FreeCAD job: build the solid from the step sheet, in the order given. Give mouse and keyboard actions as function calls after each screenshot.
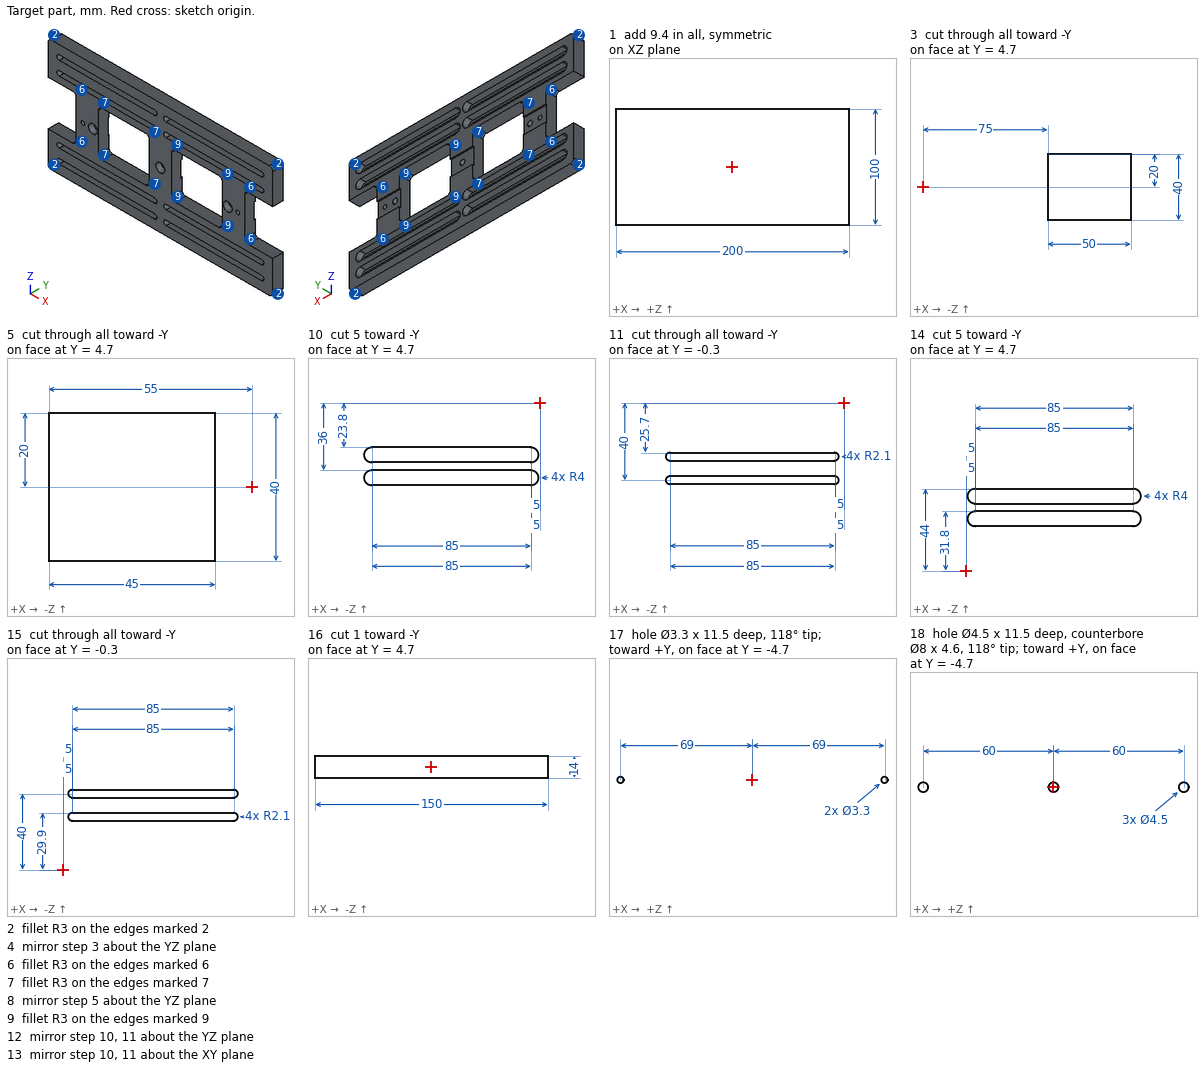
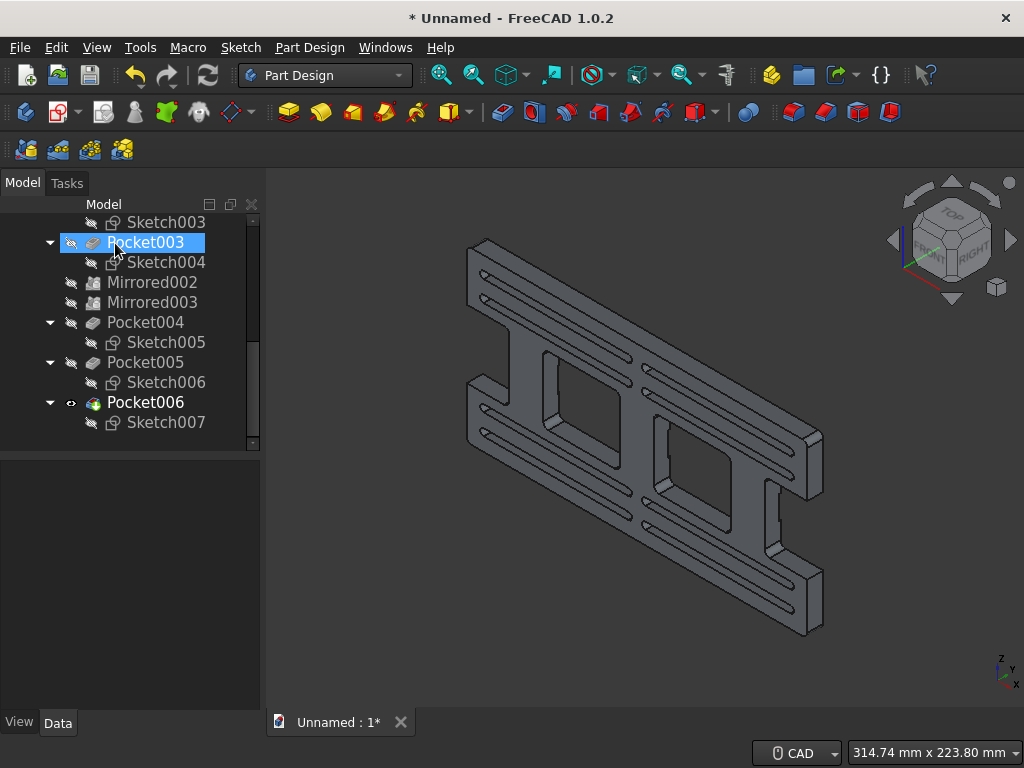
click(637, 469)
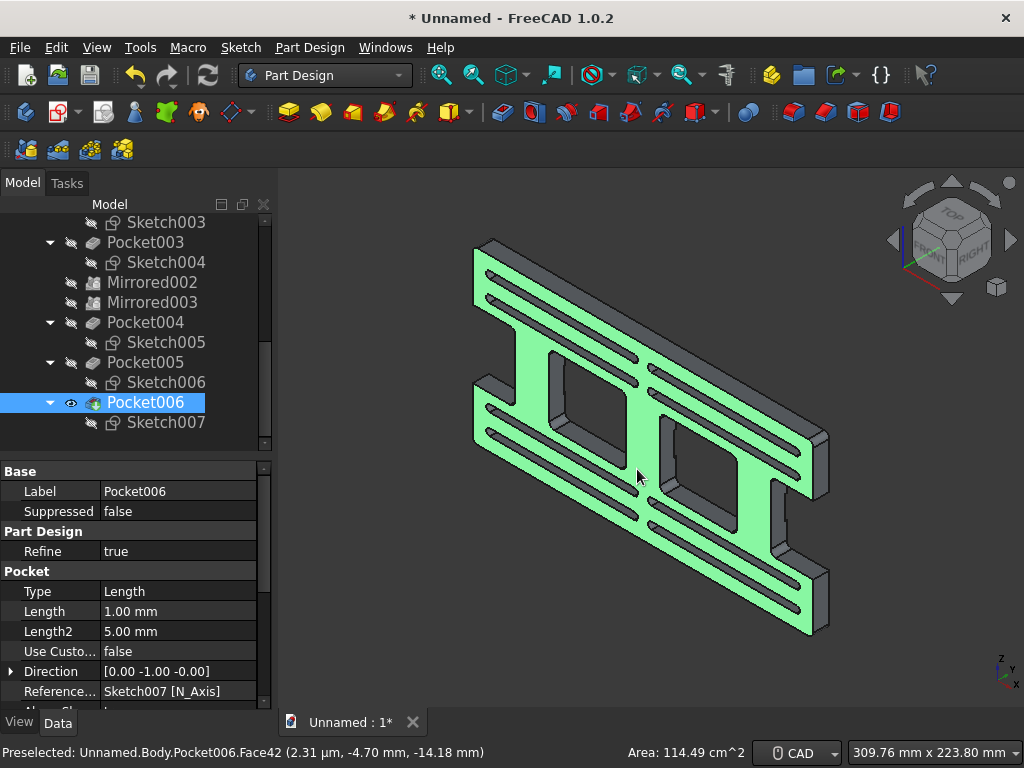
click(58, 112)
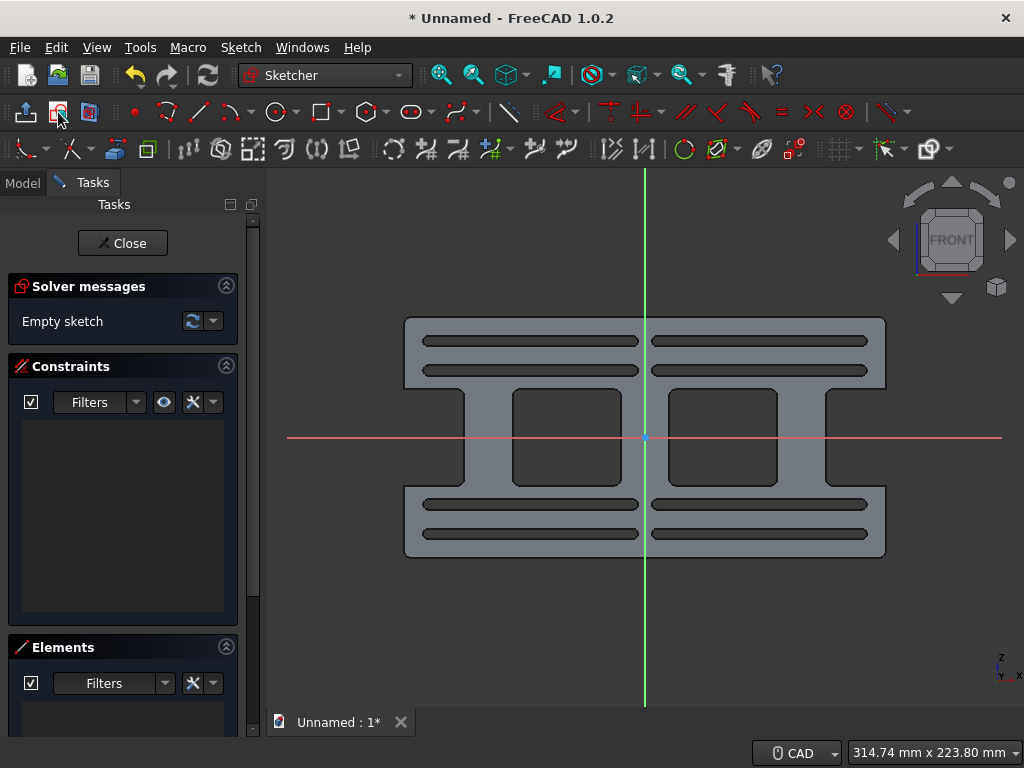
key(g)
key(c)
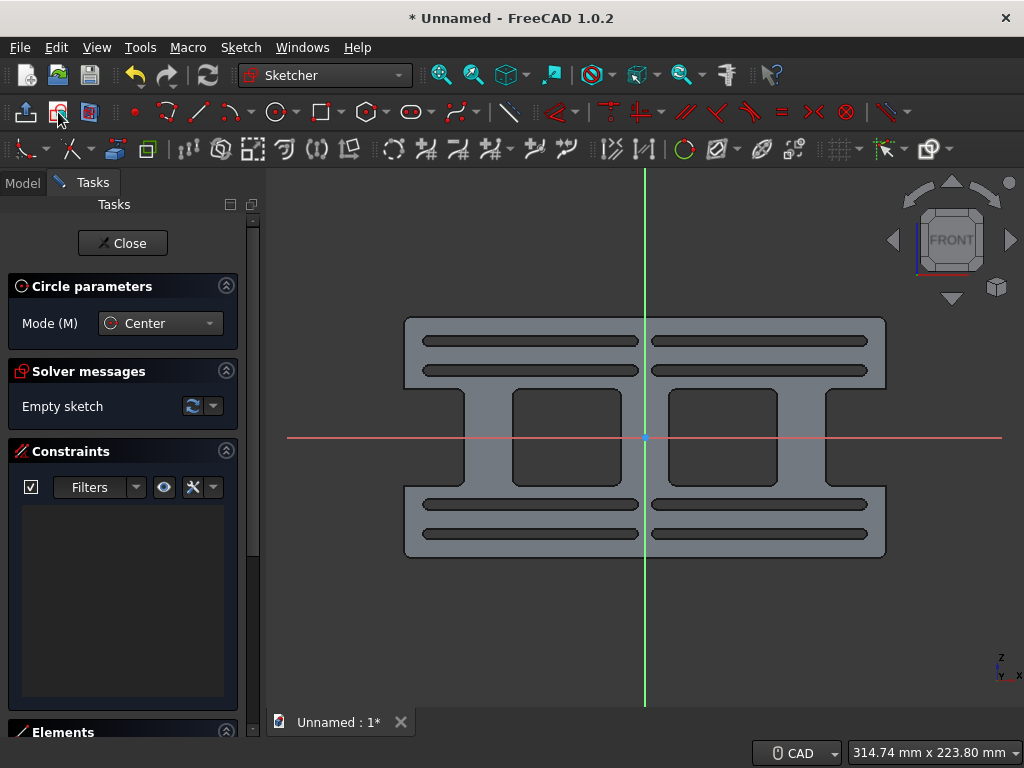
scroll(811, 438, up, 9)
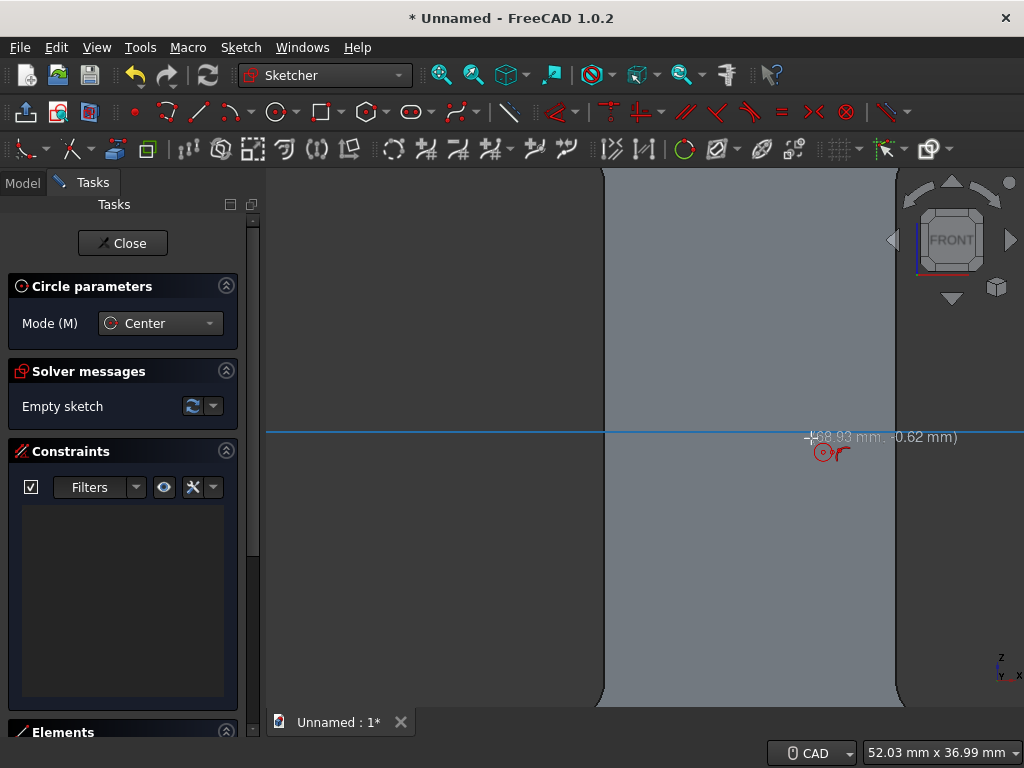
scroll(772, 439, down, 8)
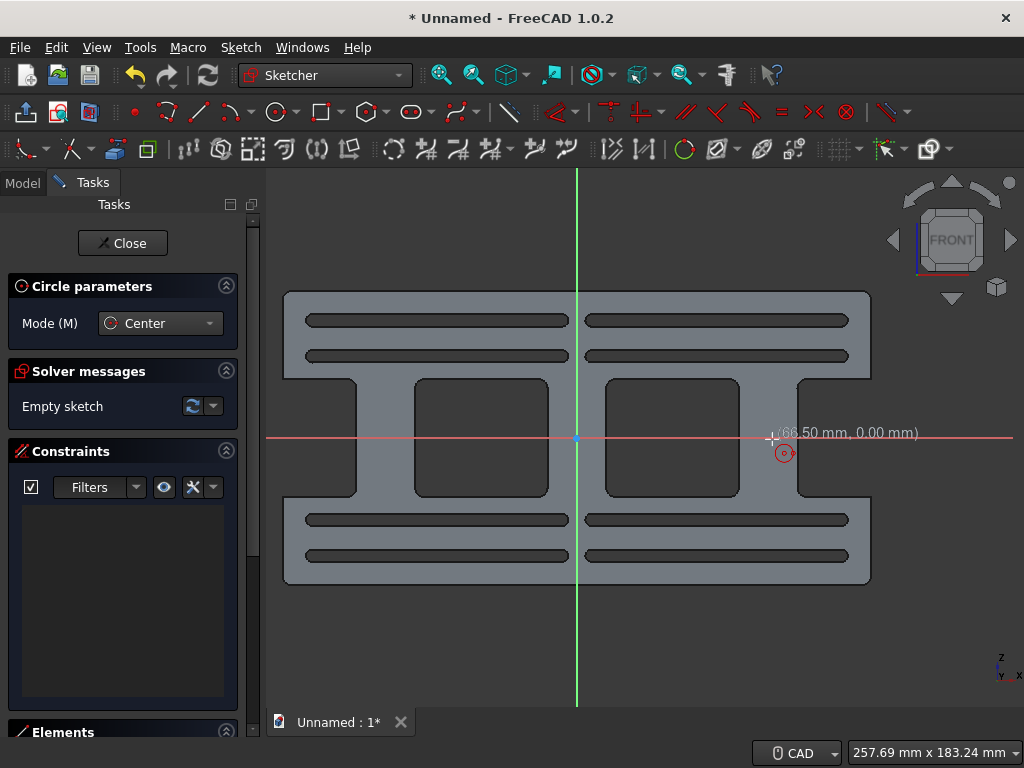
click(780, 438)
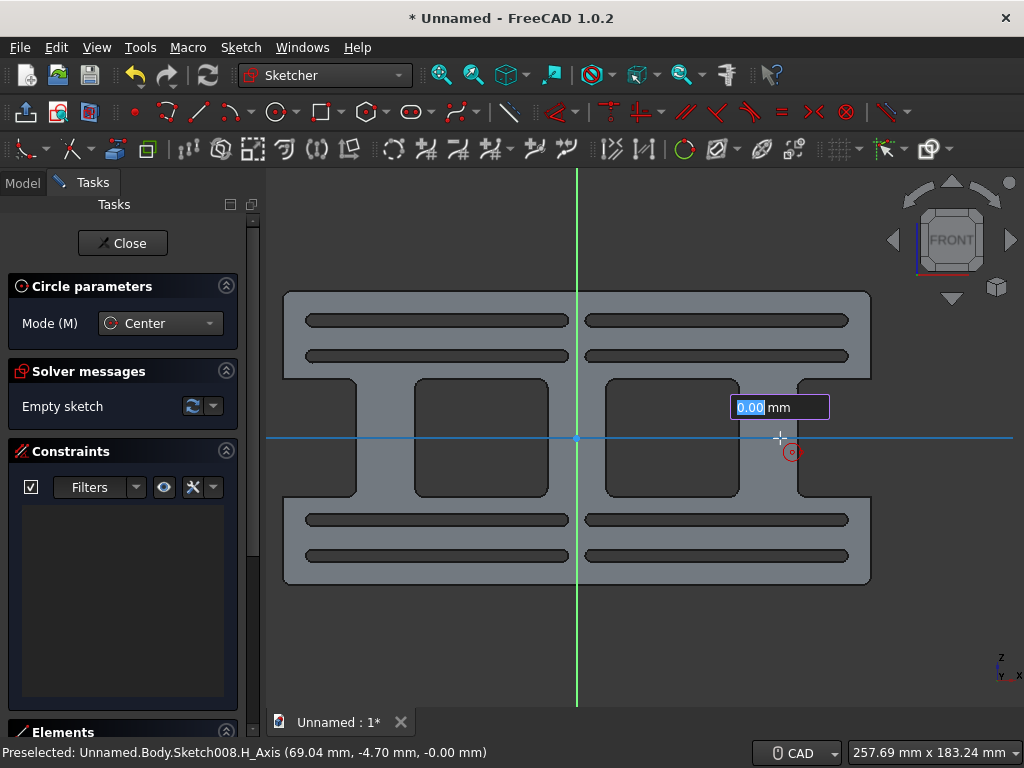
scroll(778, 443, up, 7)
move(777, 440)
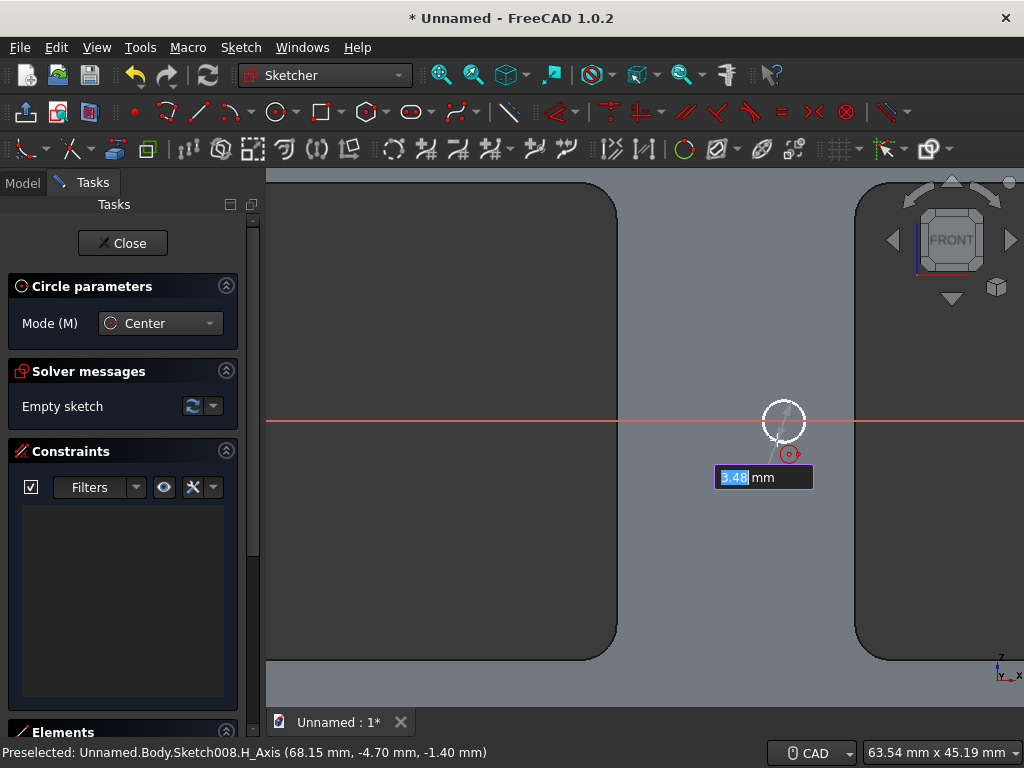
text(3.3)
key(Return)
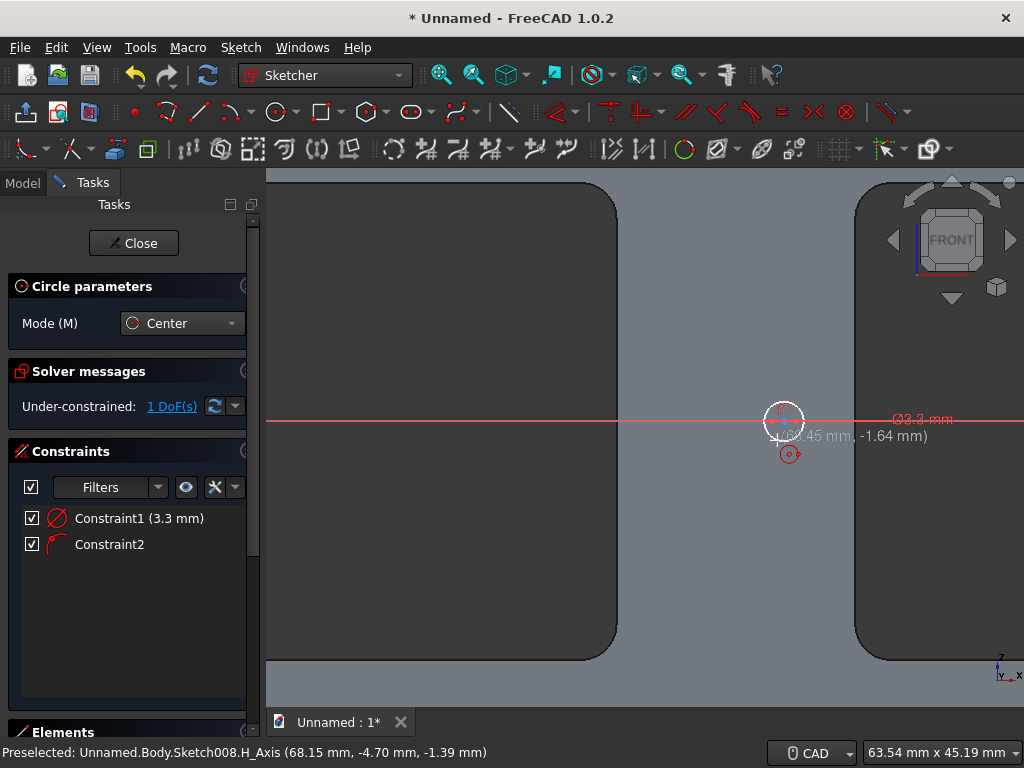
scroll(778, 443, down, 7)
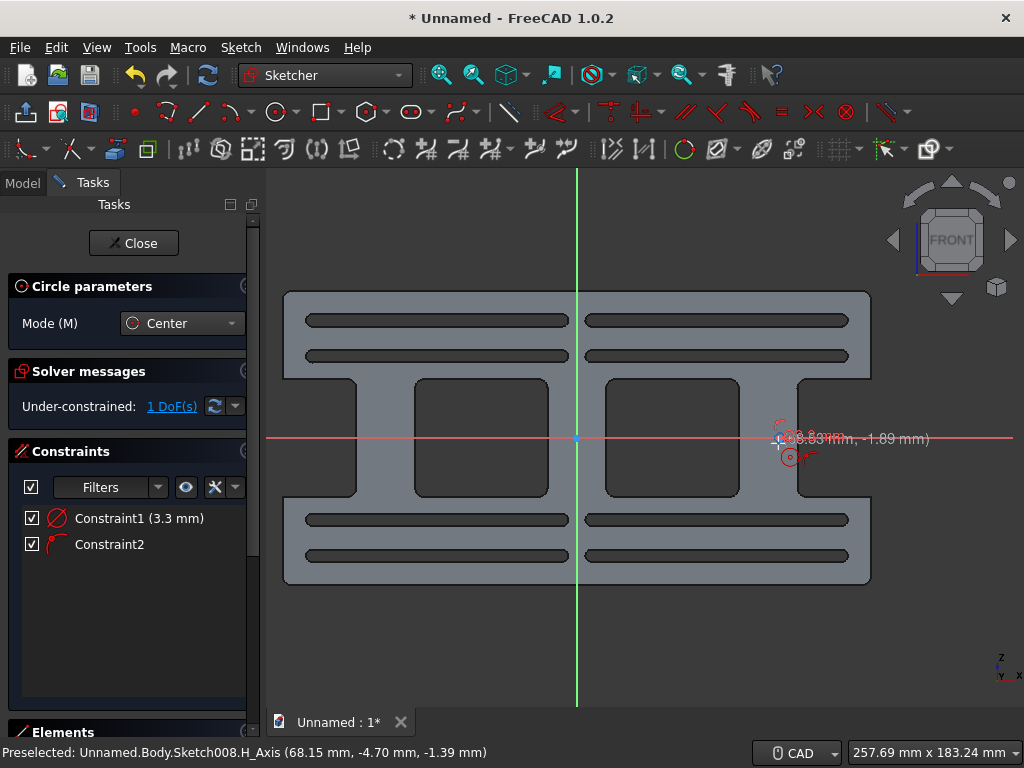
scroll(374, 438, up, 8)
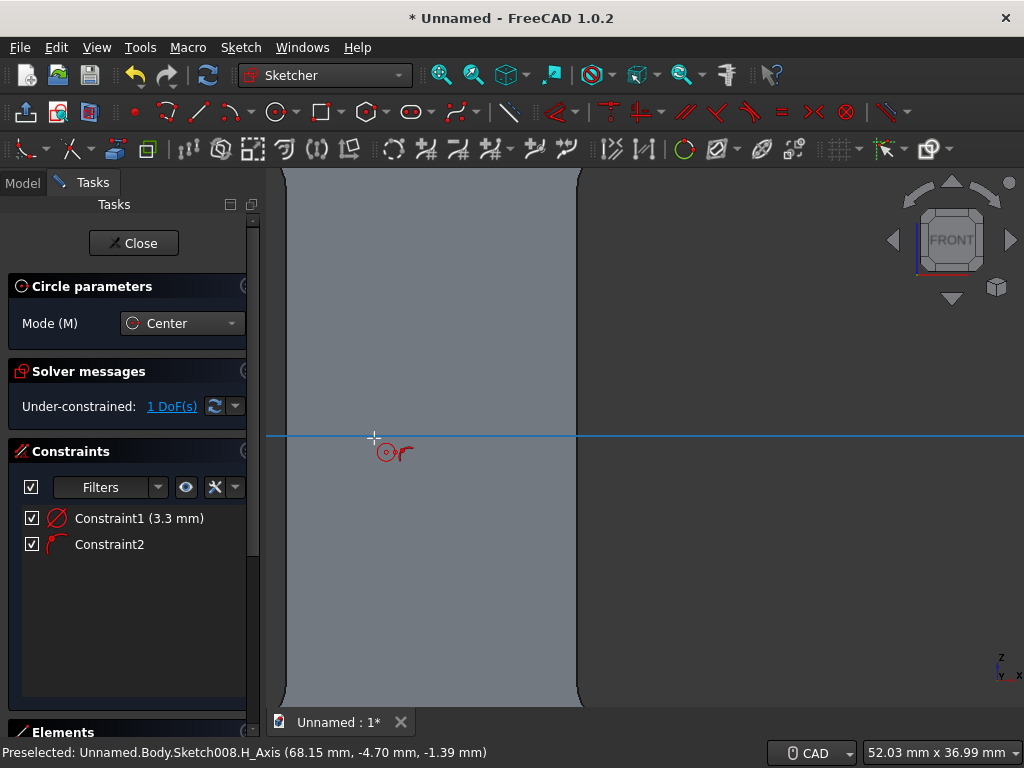
scroll(374, 438, down, 8)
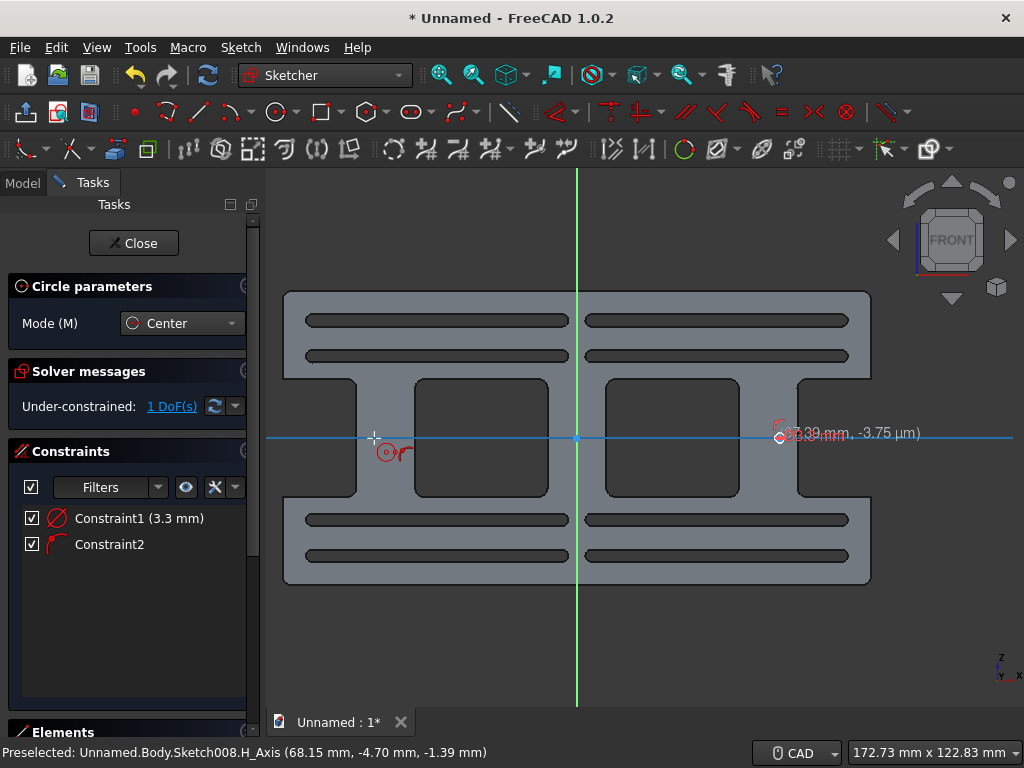
click(374, 438)